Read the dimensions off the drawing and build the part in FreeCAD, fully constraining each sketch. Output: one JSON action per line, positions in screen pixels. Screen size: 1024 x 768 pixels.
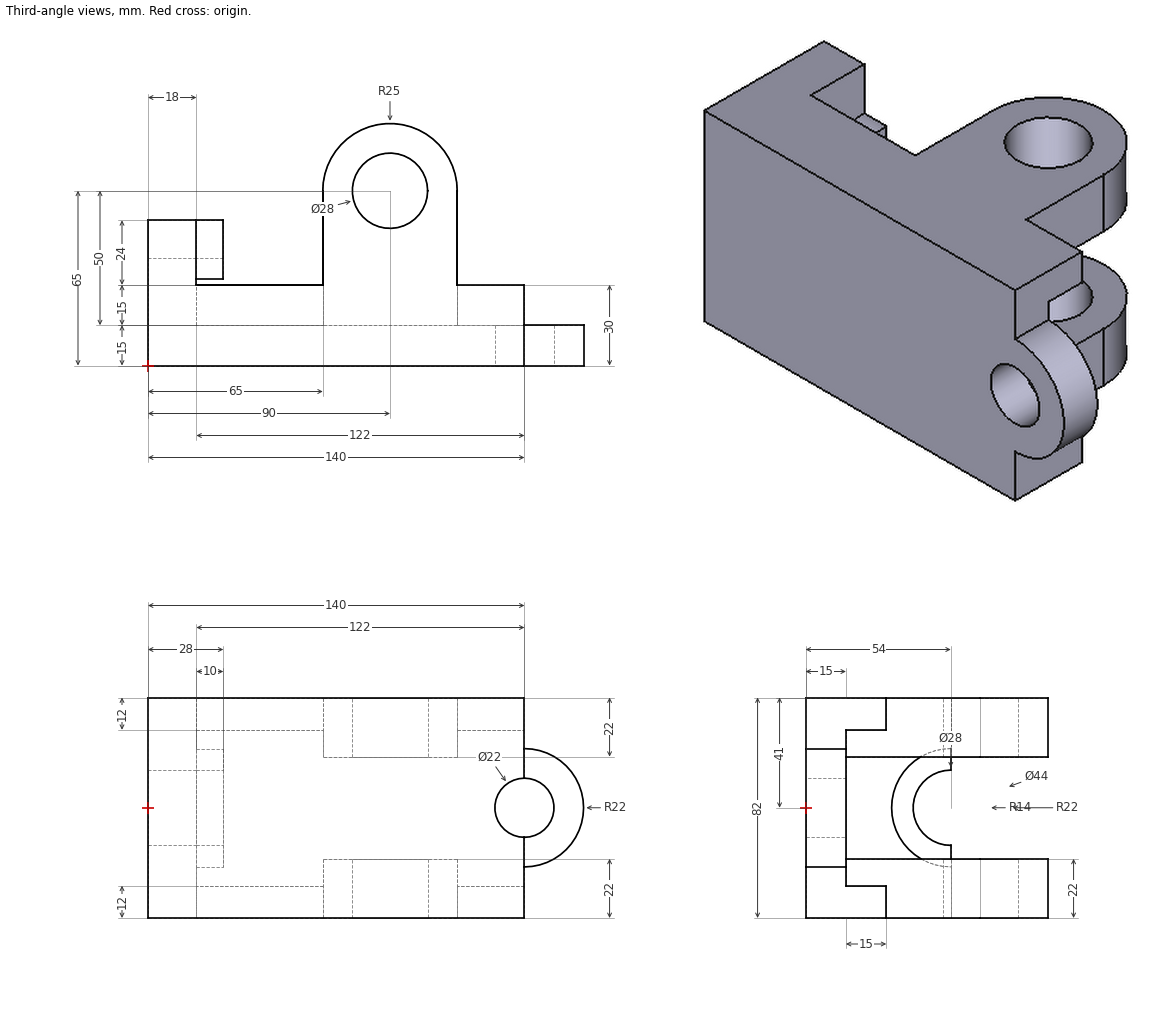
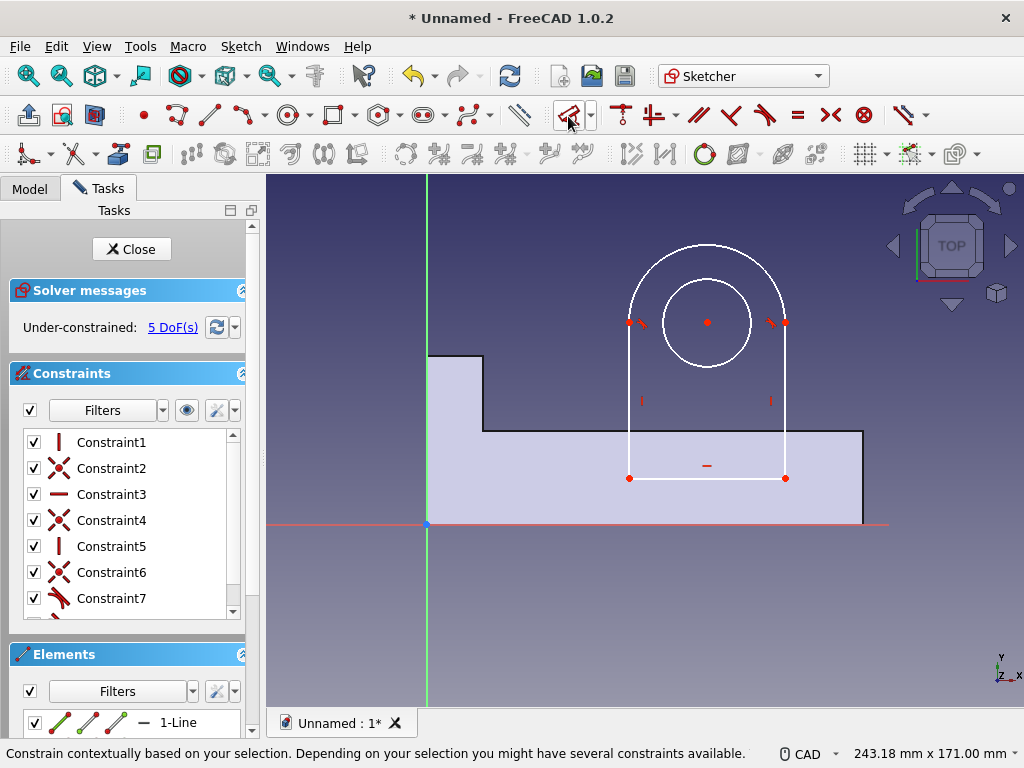
{"action": "left_click", "coordinate": [753, 260]}
{"action": "left_click", "coordinate": [772, 234]}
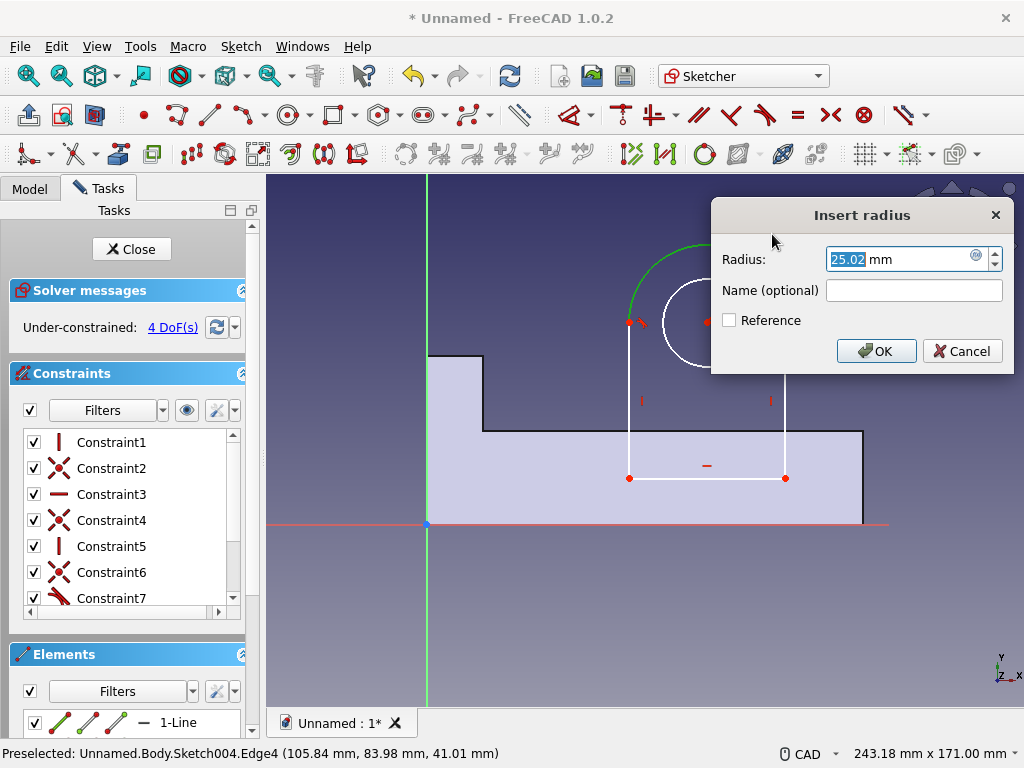
{"action": "type", "text": "25"}
{"action": "key", "text": "Return"}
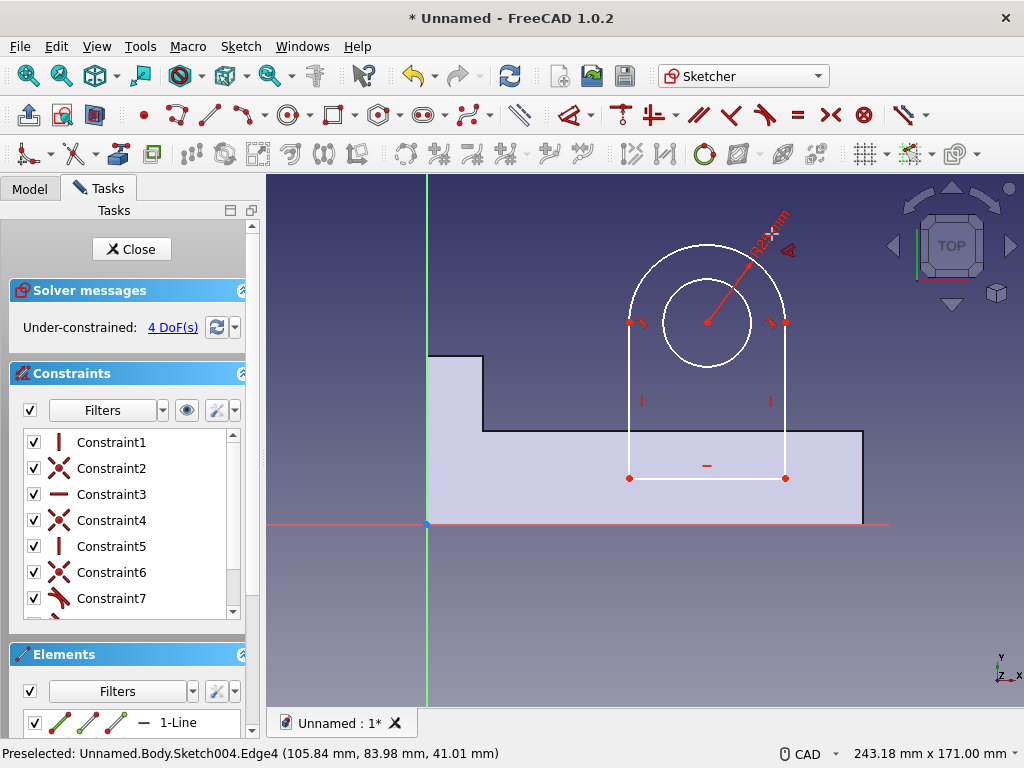
{"action": "left_click", "coordinate": [738, 292]}
{"action": "left_click", "coordinate": [761, 376]}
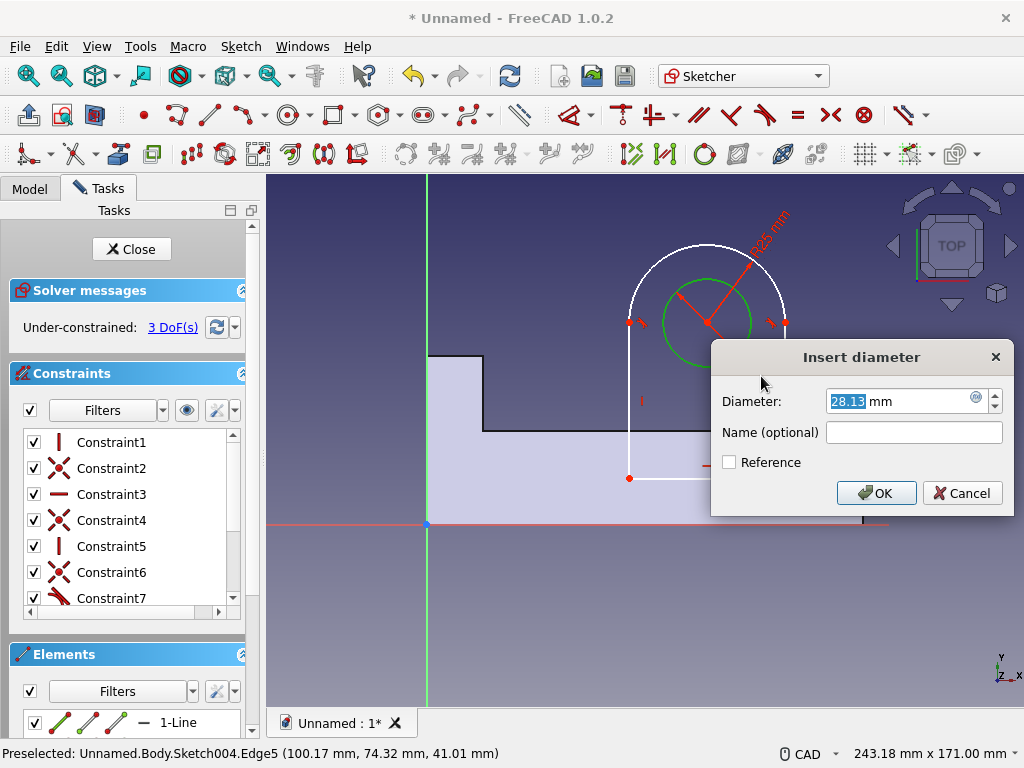
{"action": "type", "text": "28"}
{"action": "key", "text": "Return"}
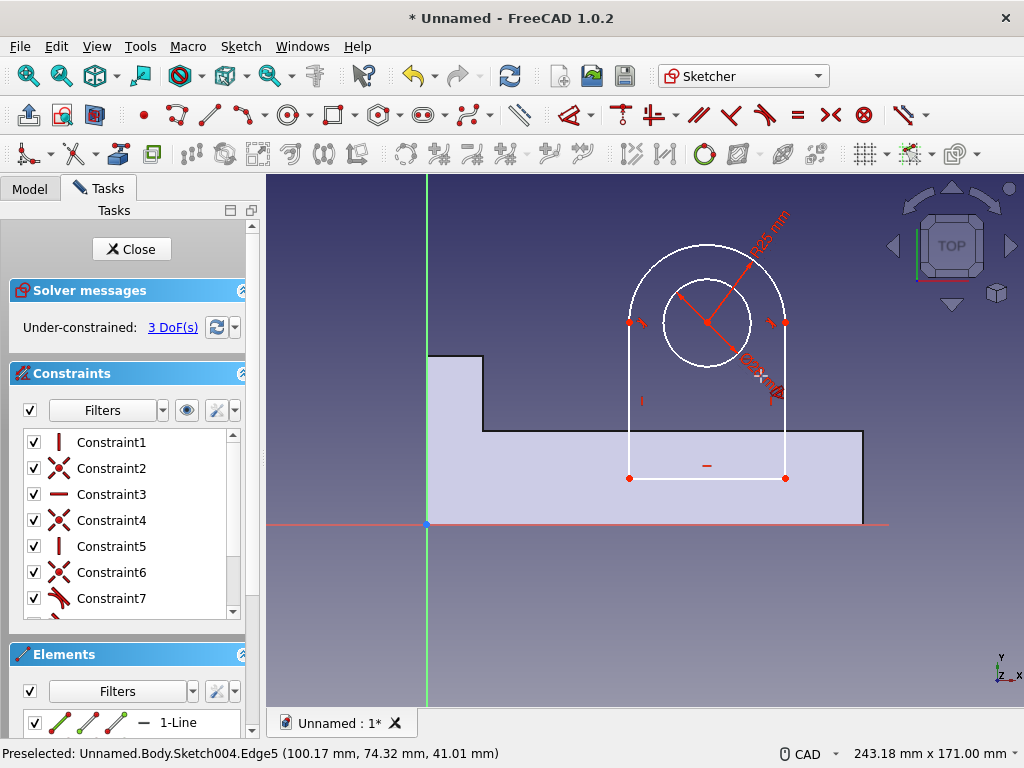
{"action": "left_click", "coordinate": [629, 370]}
{"action": "left_click", "coordinate": [663, 401]}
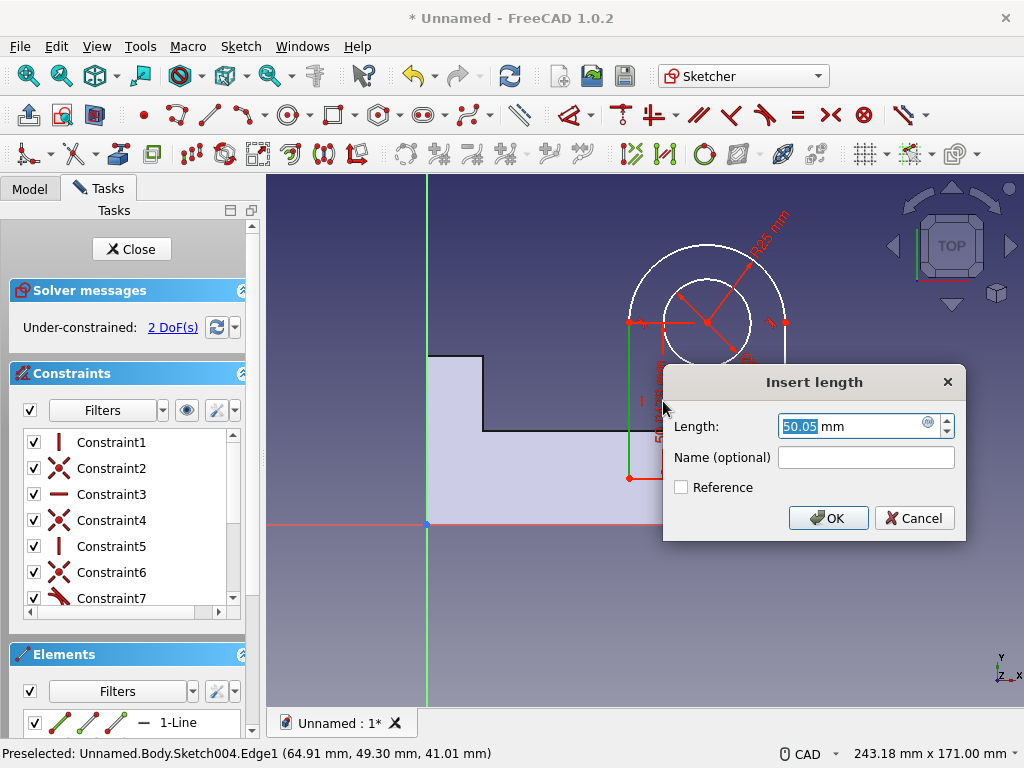
{"action": "type", "text": "50"}
{"action": "key", "text": "Return"}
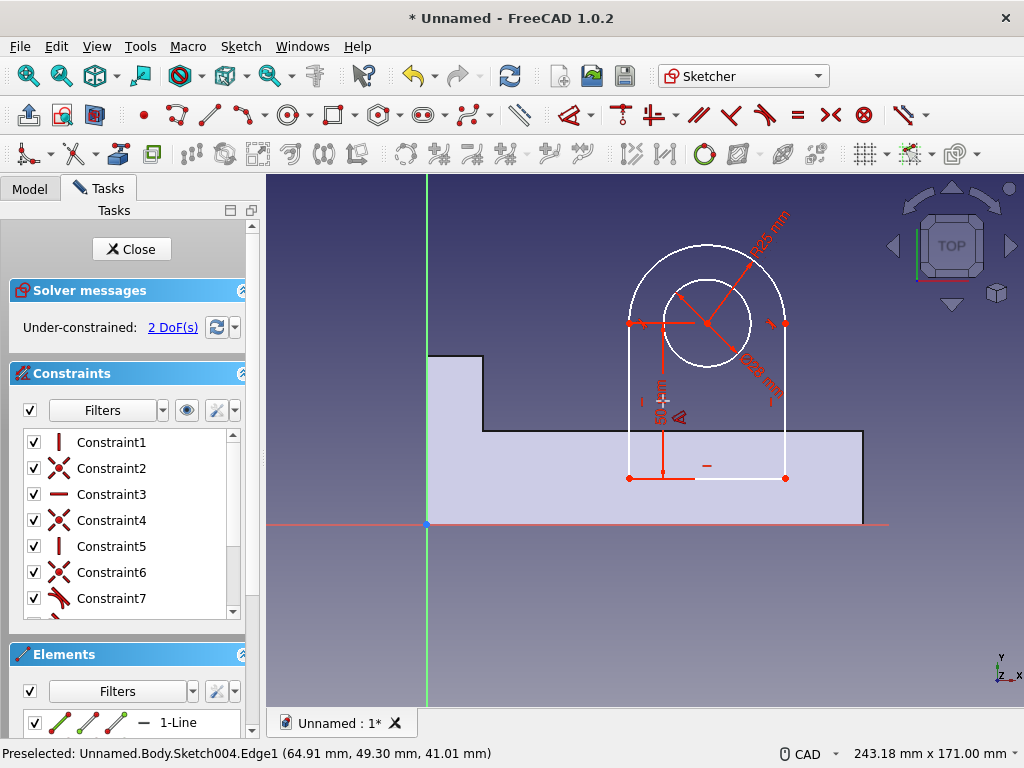
{"action": "left_click", "coordinate": [707, 323]}
{"action": "left_click", "coordinate": [567, 559]}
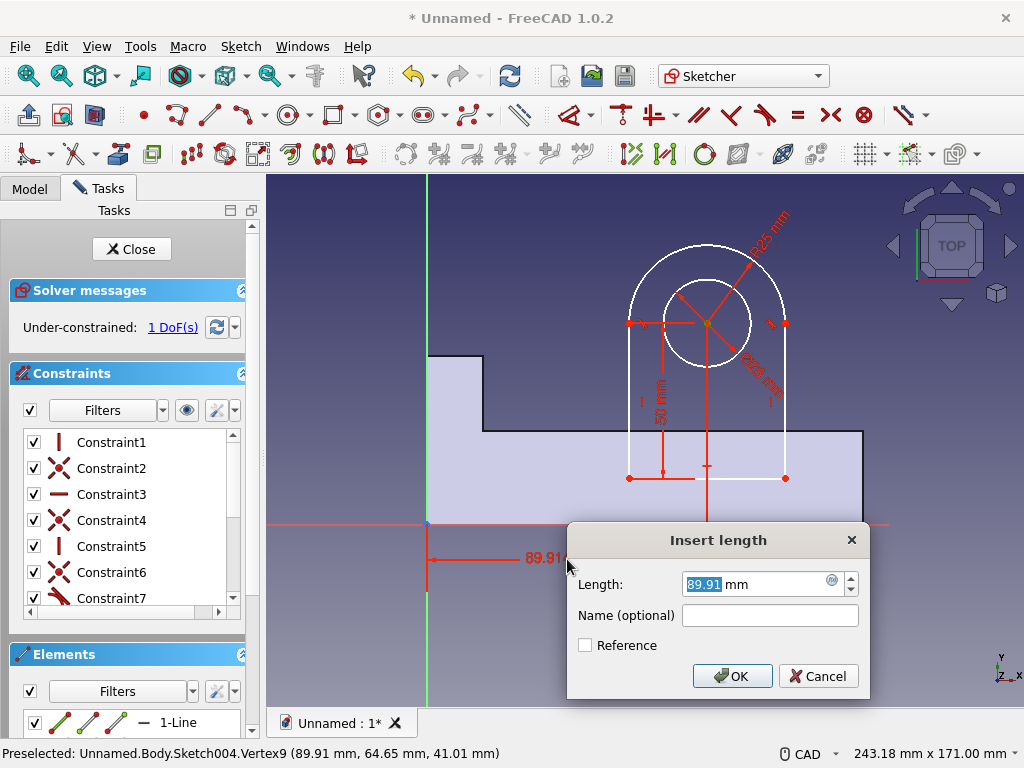
{"action": "type", "text": "90"}
{"action": "key", "text": "Return"}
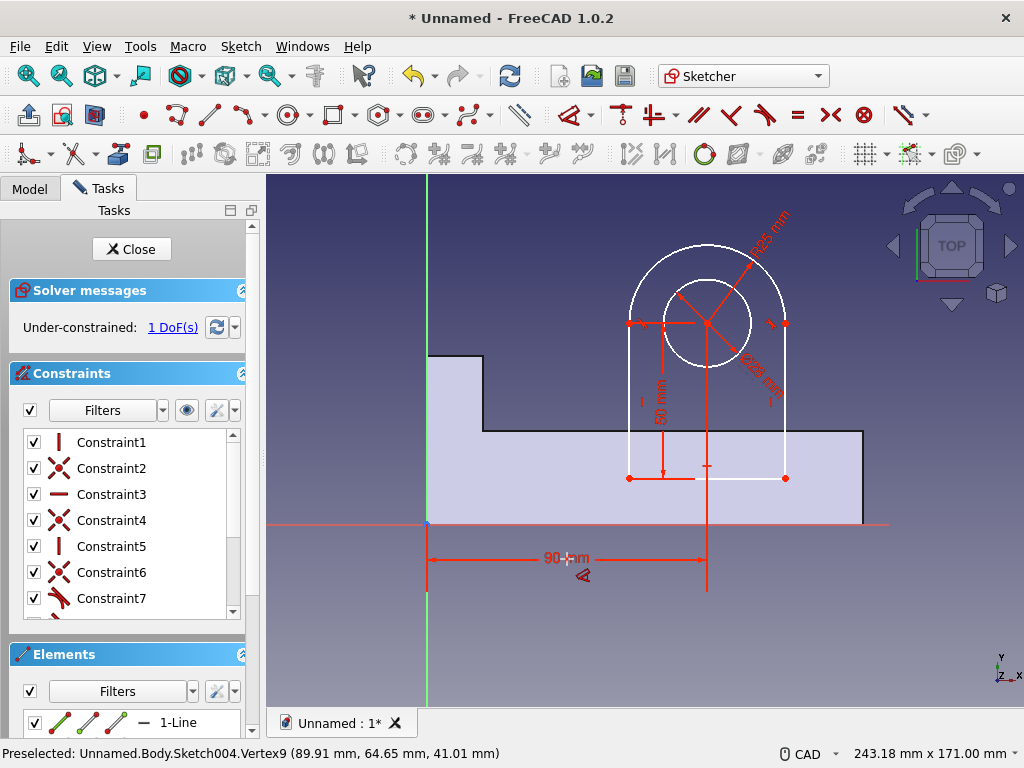
{"action": "left_click", "coordinate": [707, 323]}
{"action": "left_click", "coordinate": [393, 424]}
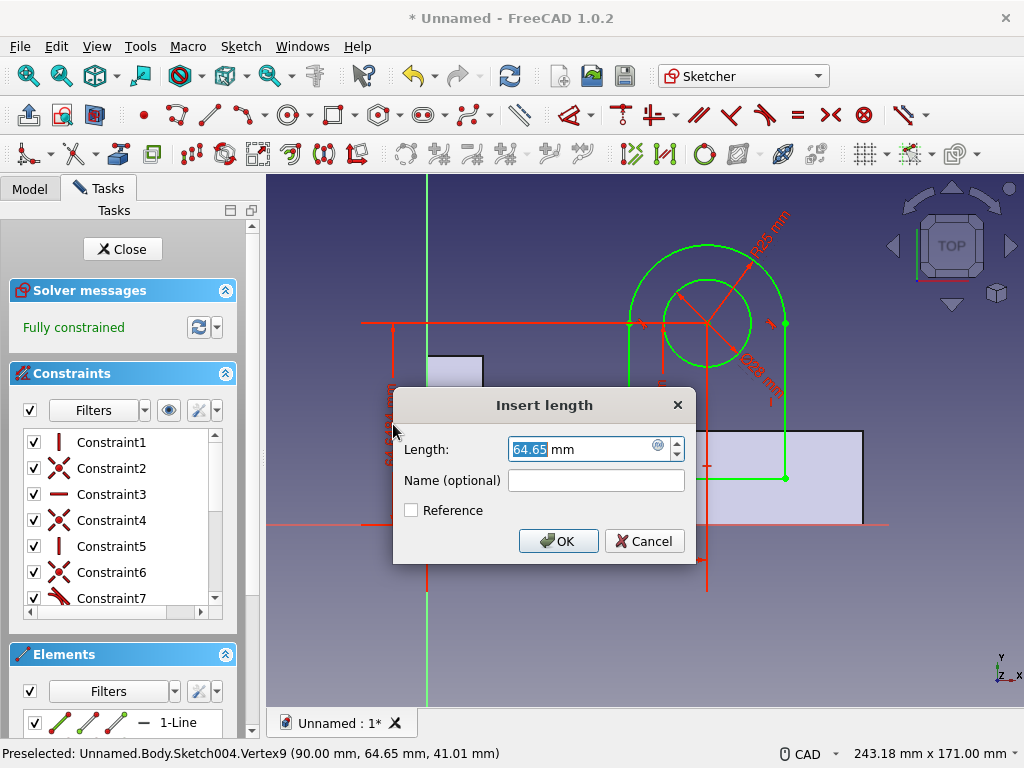
{"action": "type", "text": "65"}
{"action": "key", "text": "Return"}
{"action": "key", "text": "Escape"}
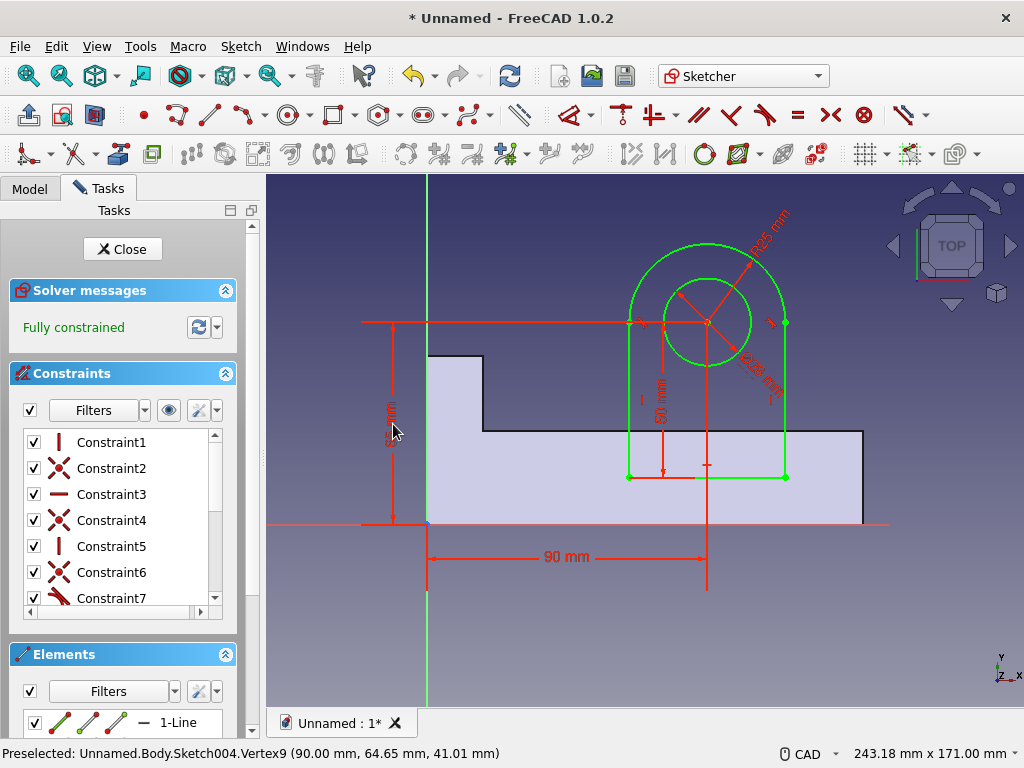
{"action": "left_click", "coordinate": [123, 249]}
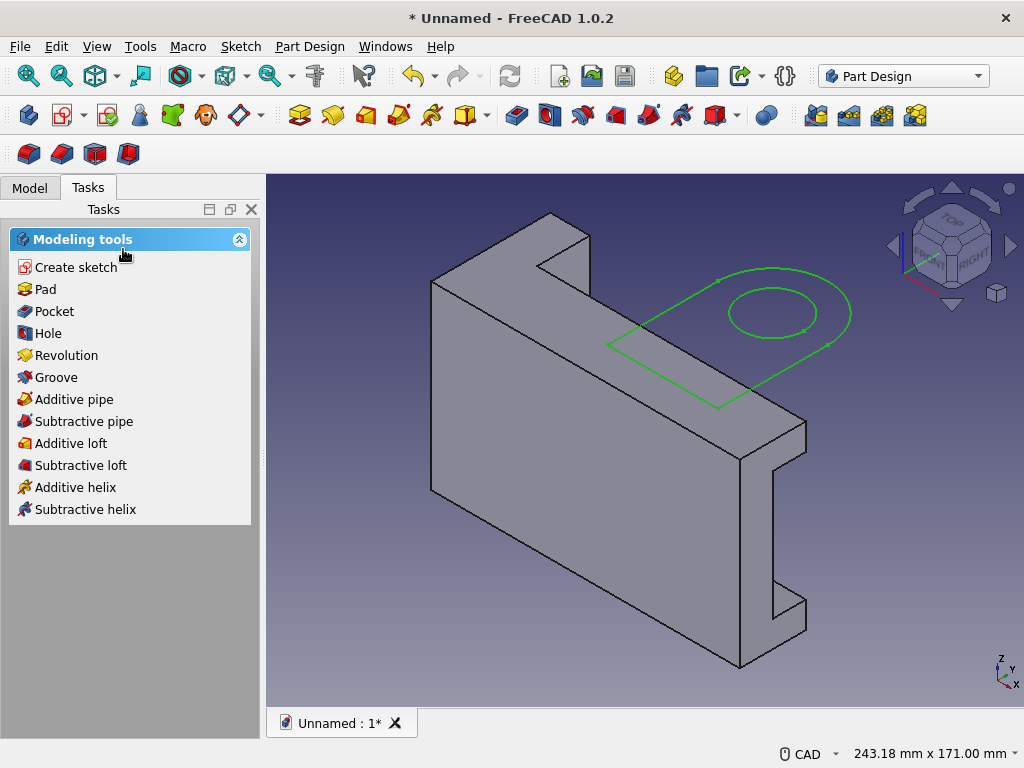
{"action": "left_click", "coordinate": [300, 116]}